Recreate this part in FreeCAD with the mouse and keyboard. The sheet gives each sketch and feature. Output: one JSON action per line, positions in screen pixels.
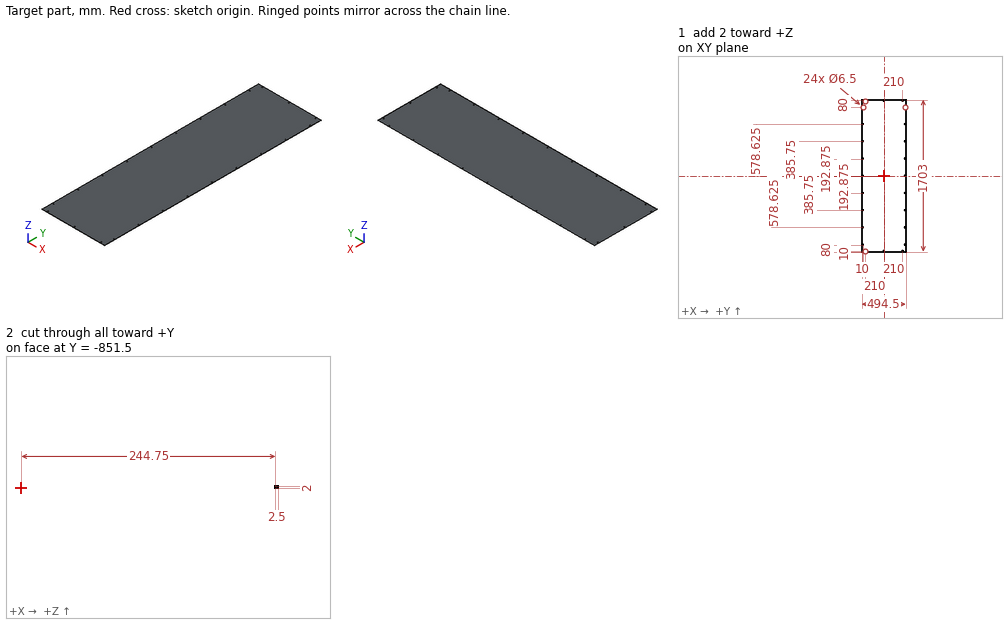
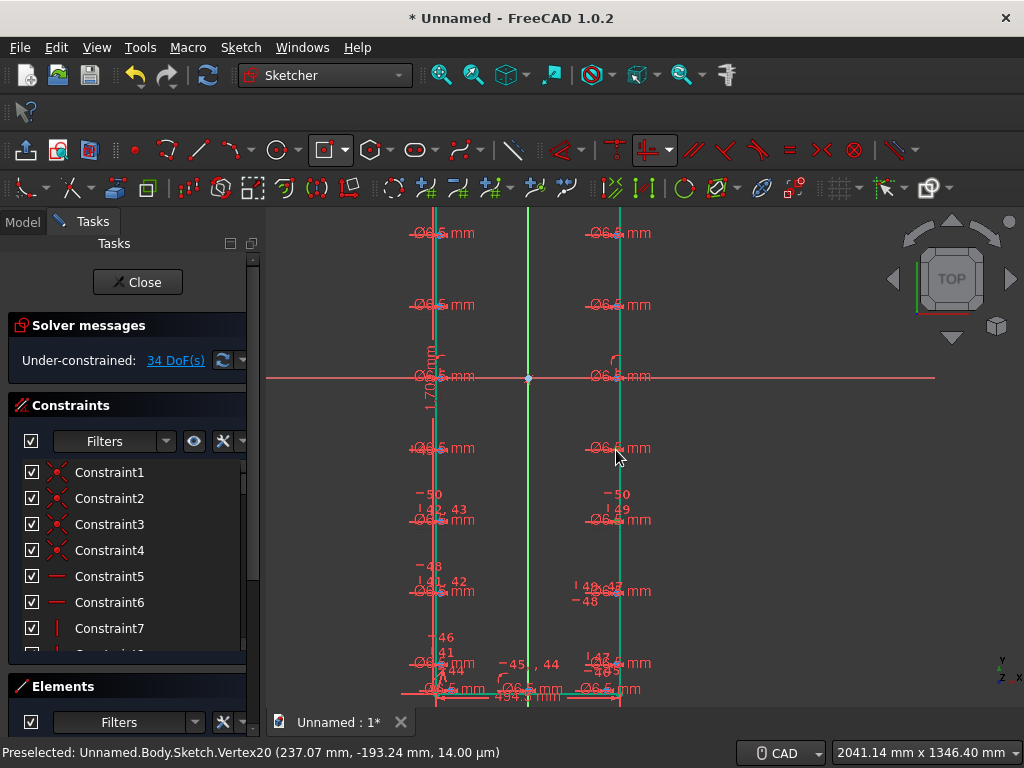
{"action": "left_click", "coordinate": [672, 150]}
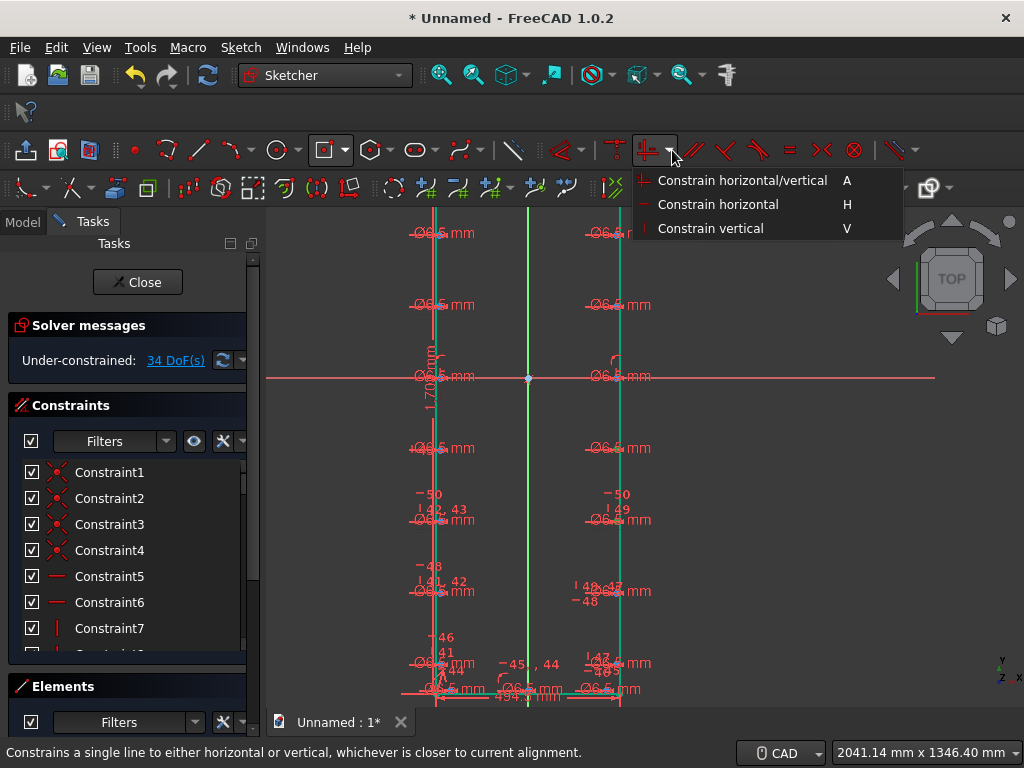
{"action": "left_click", "coordinate": [768, 228]}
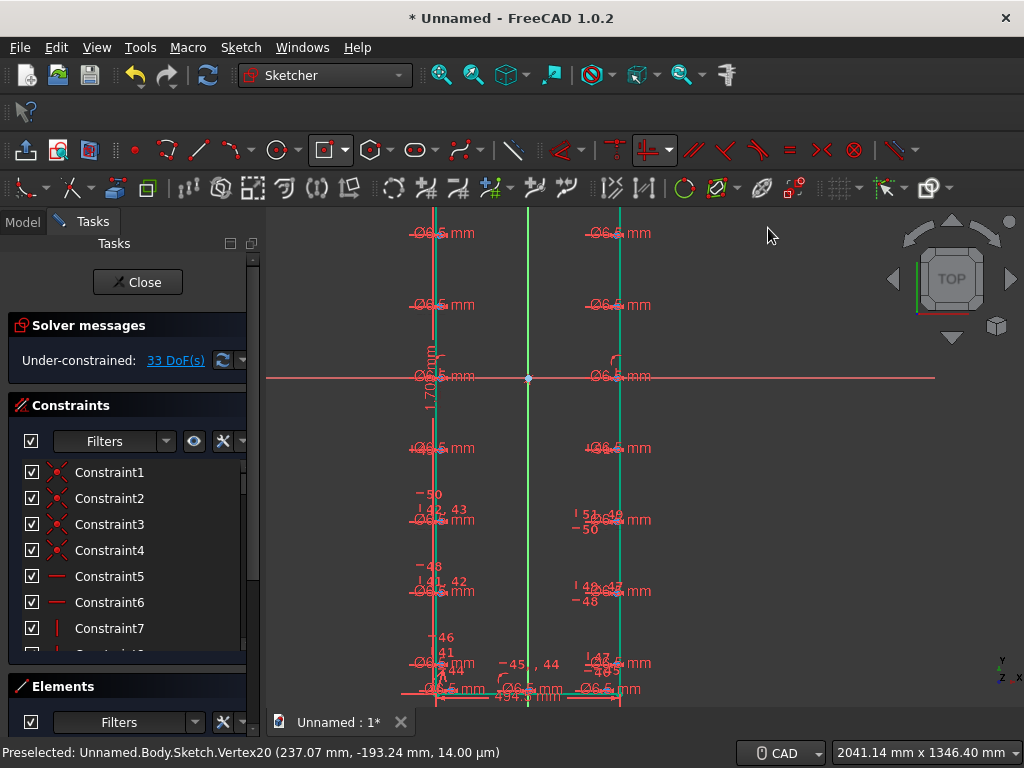
{"action": "left_click", "coordinate": [440, 450]}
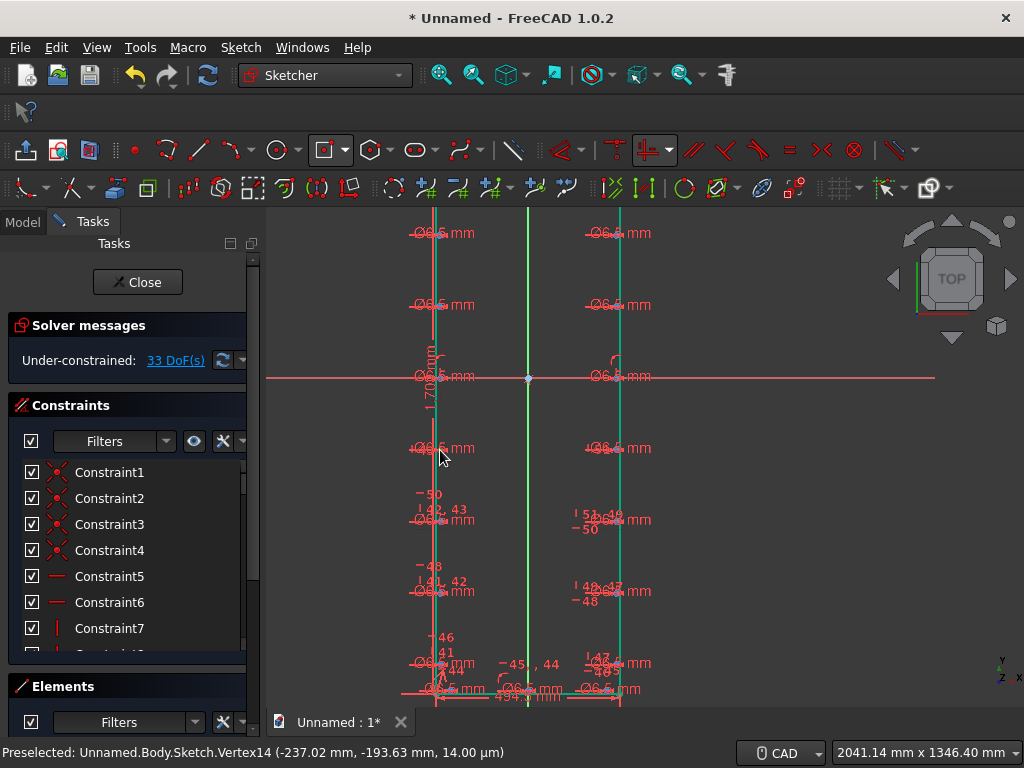
{"action": "left_click", "coordinate": [616, 450]}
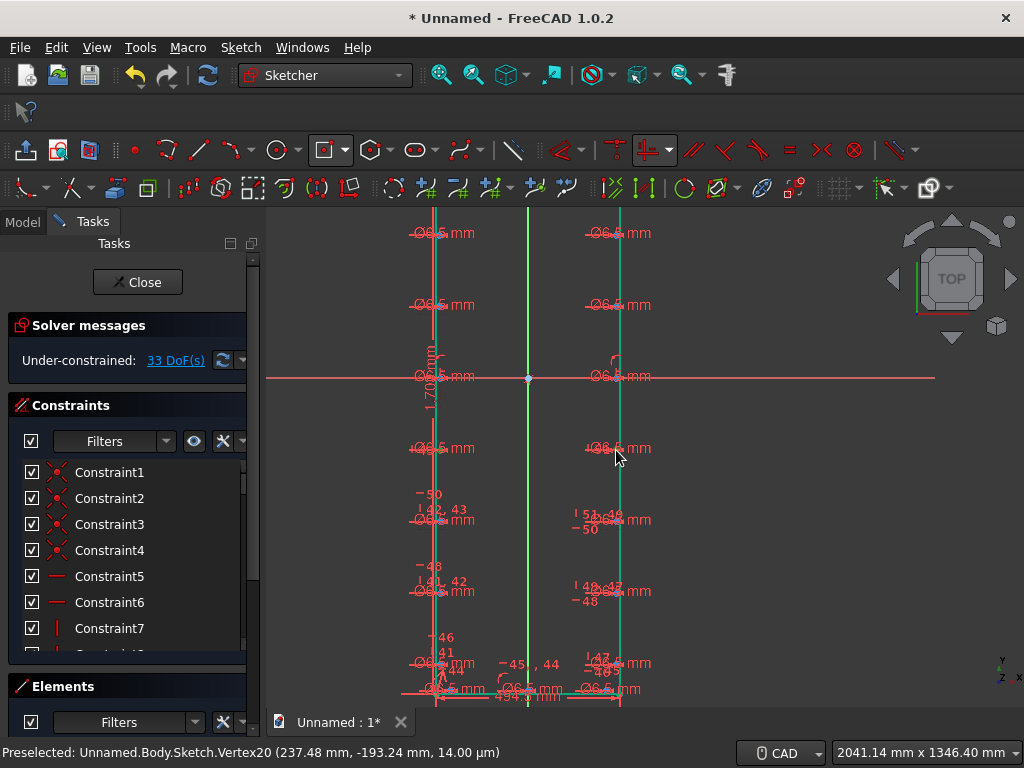
{"action": "left_click", "coordinate": [672, 150]}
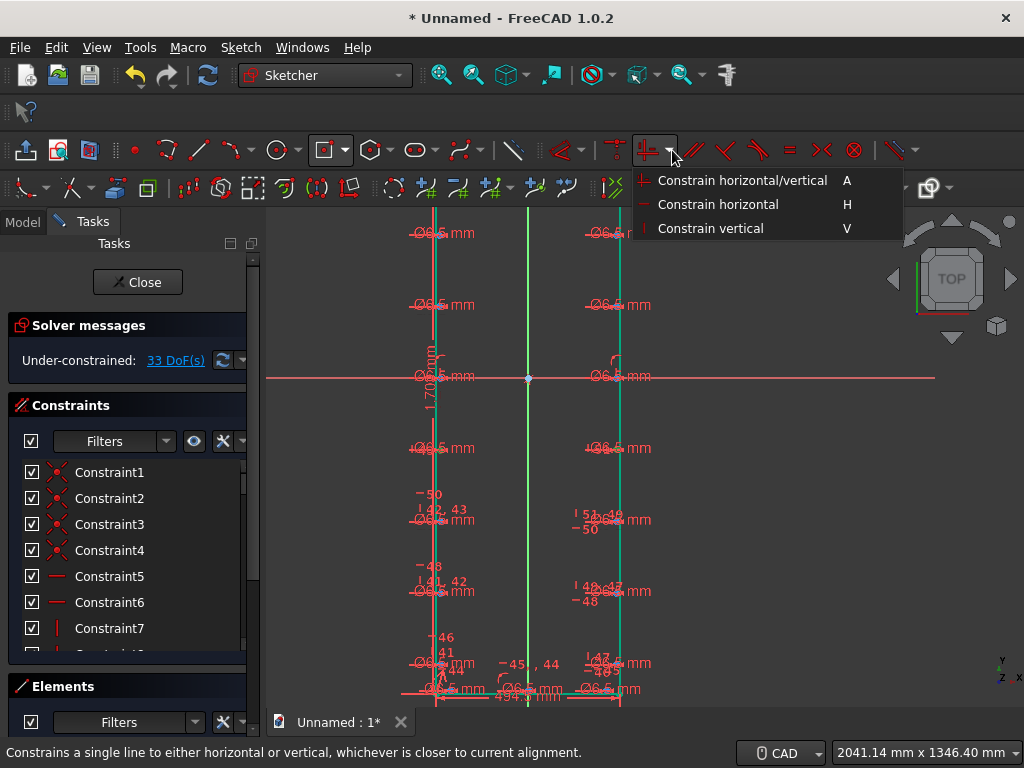
{"action": "left_click", "coordinate": [768, 204]}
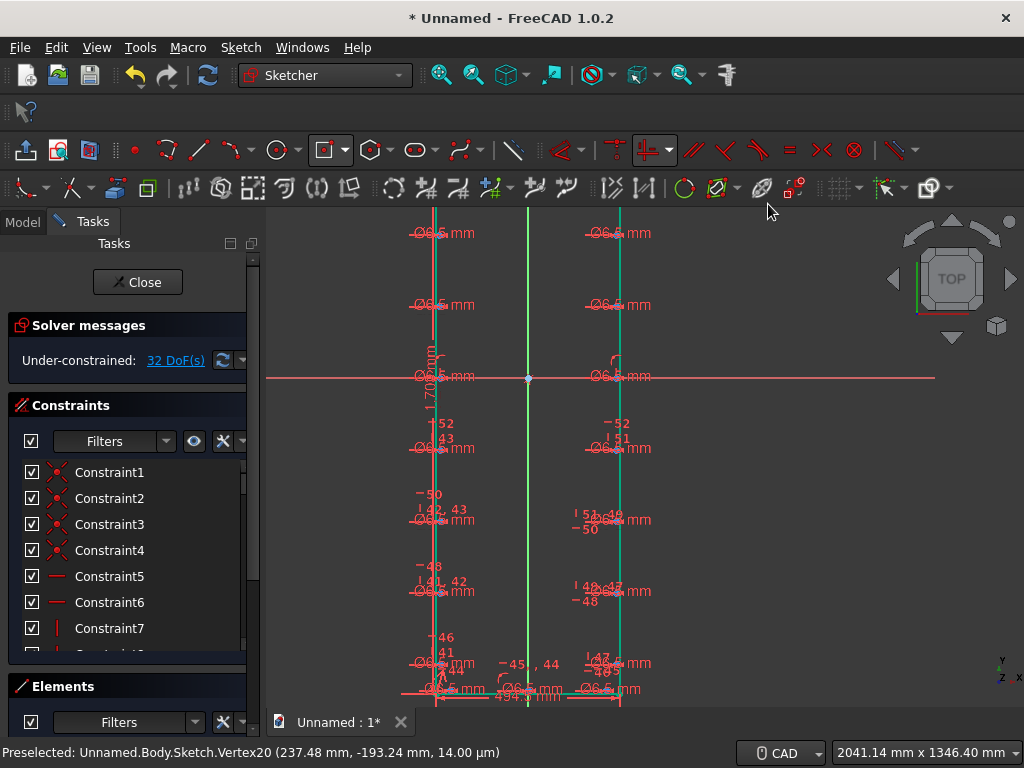
{"action": "left_click", "coordinate": [440, 450]}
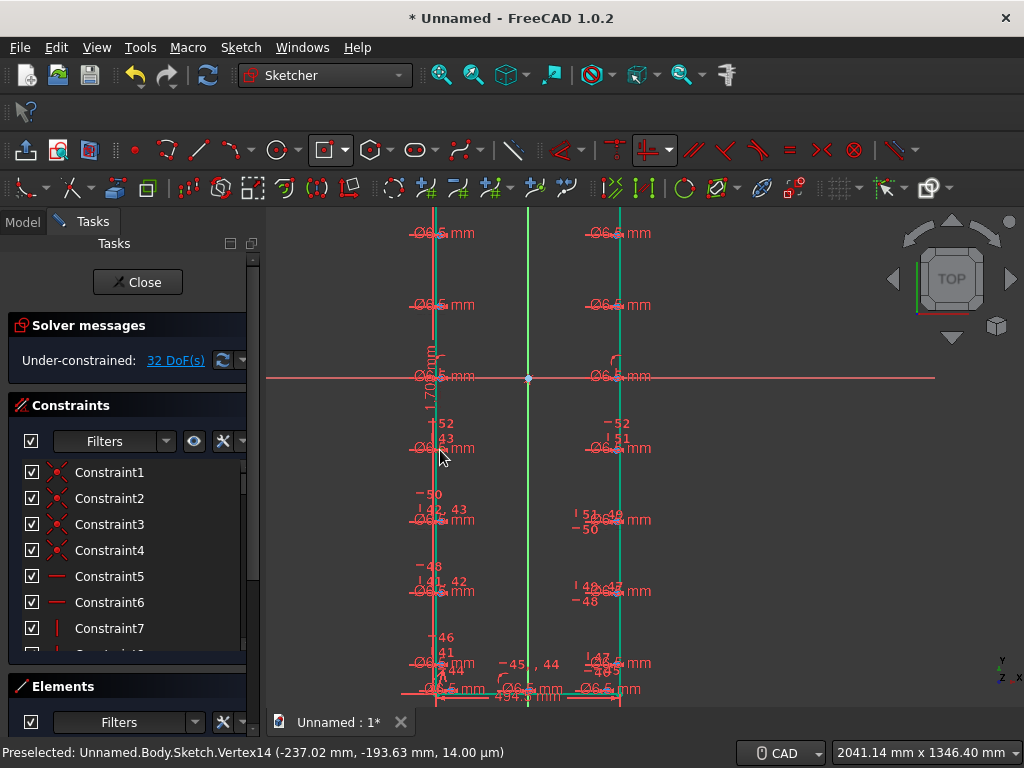
{"action": "left_click", "coordinate": [440, 378]}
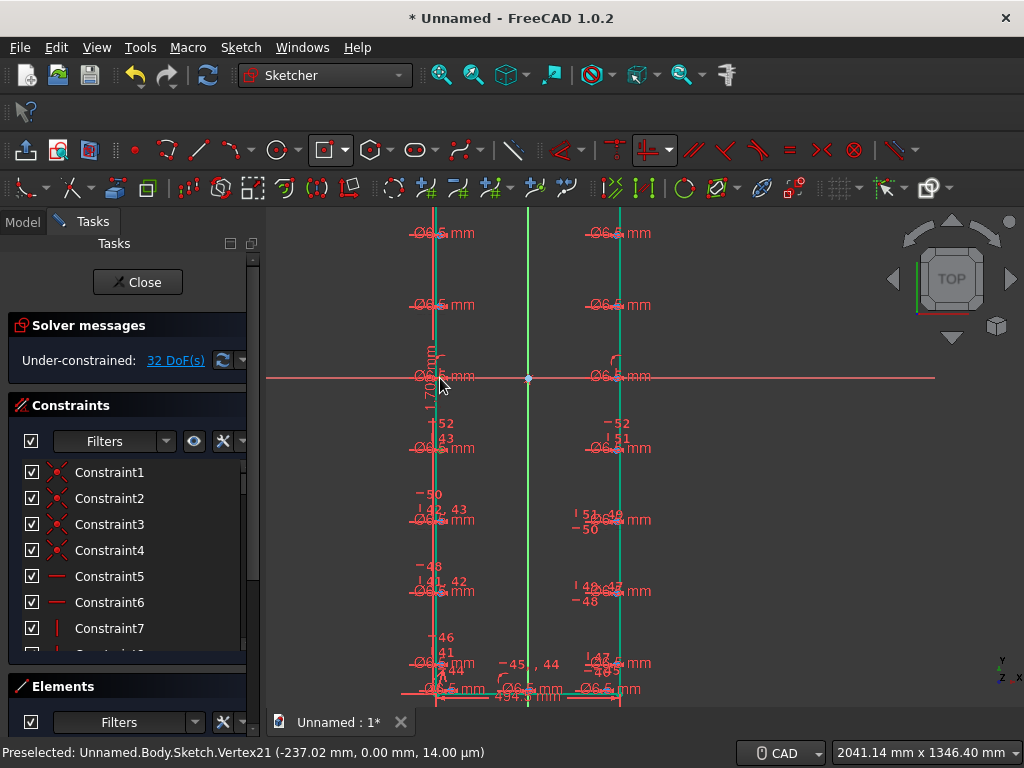
{"action": "left_click", "coordinate": [672, 150]}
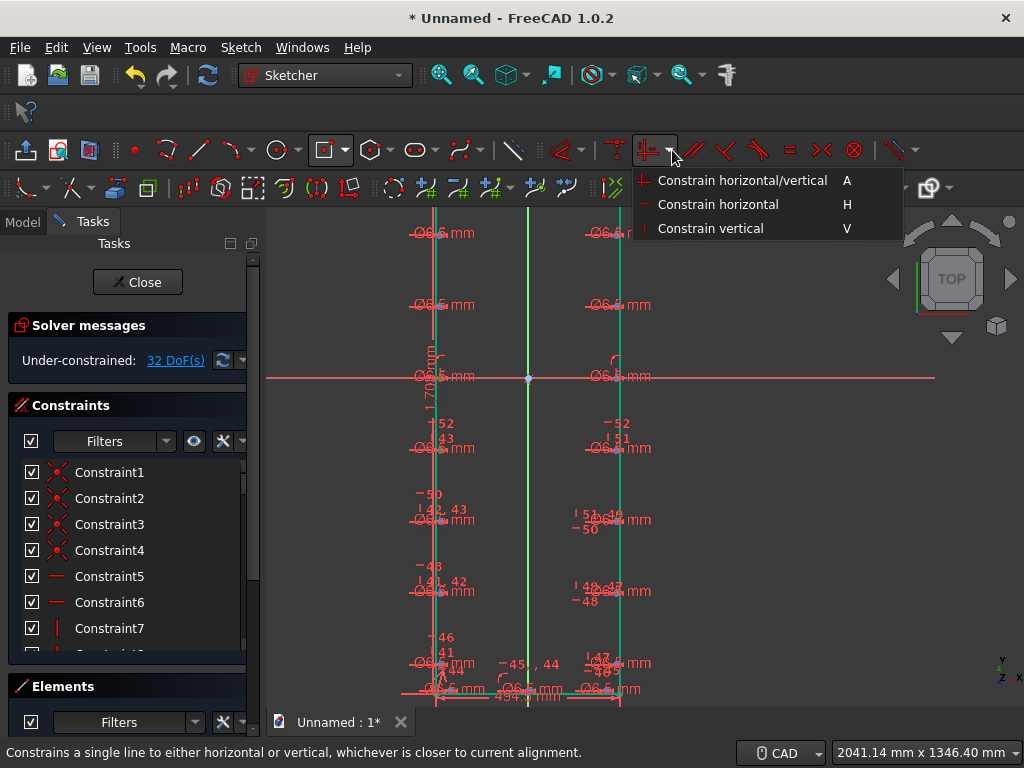
{"action": "left_click", "coordinate": [768, 228]}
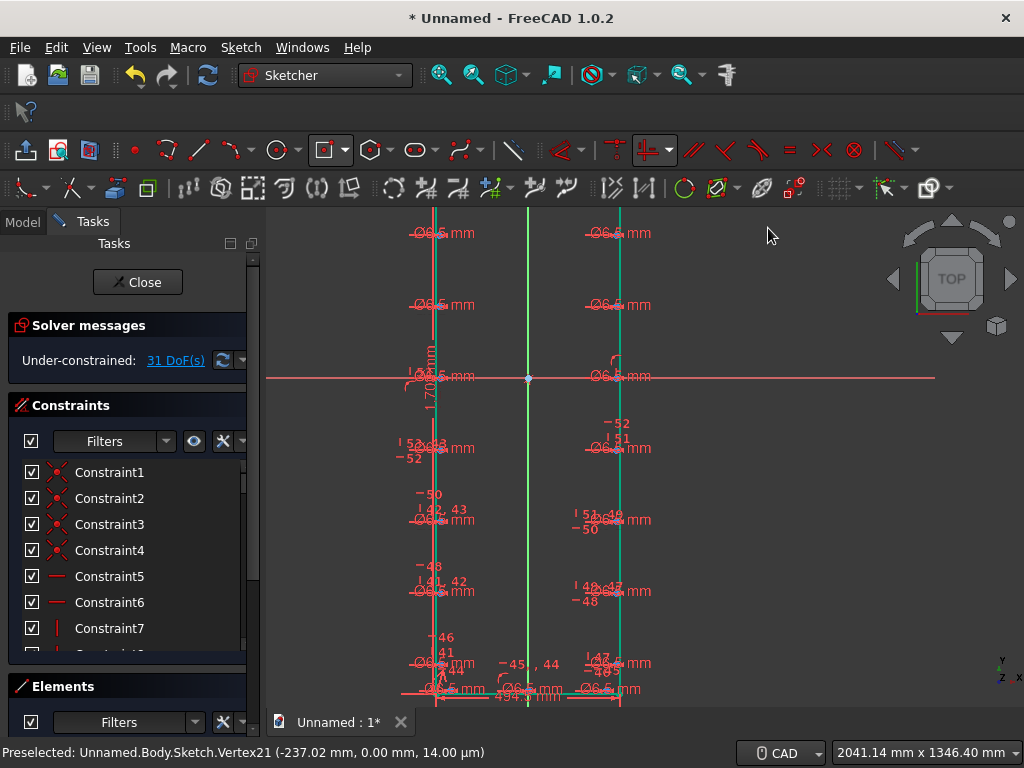
{"action": "left_click", "coordinate": [440, 378]}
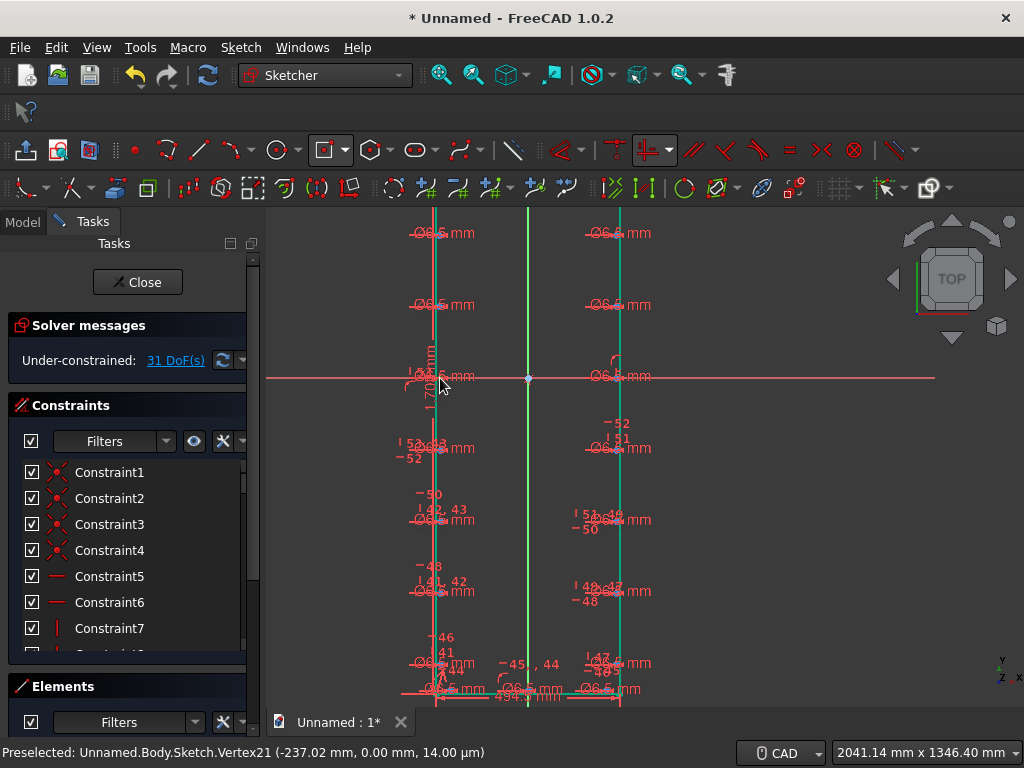
{"action": "left_click", "coordinate": [440, 307]}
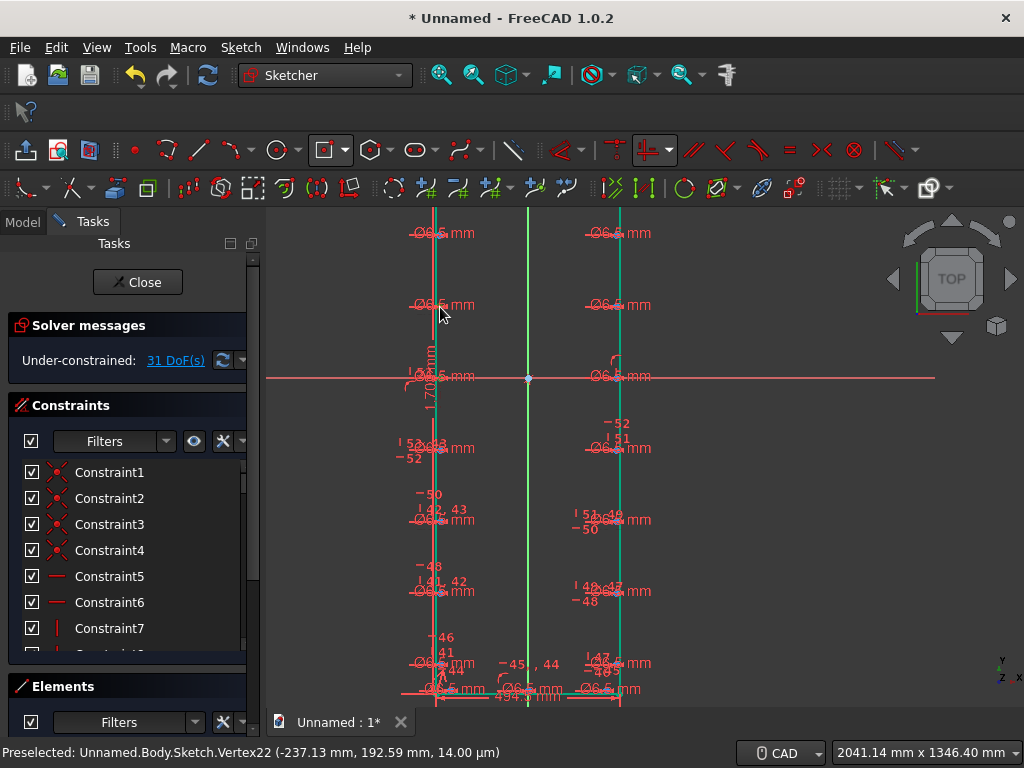
{"action": "key", "text": "v"}